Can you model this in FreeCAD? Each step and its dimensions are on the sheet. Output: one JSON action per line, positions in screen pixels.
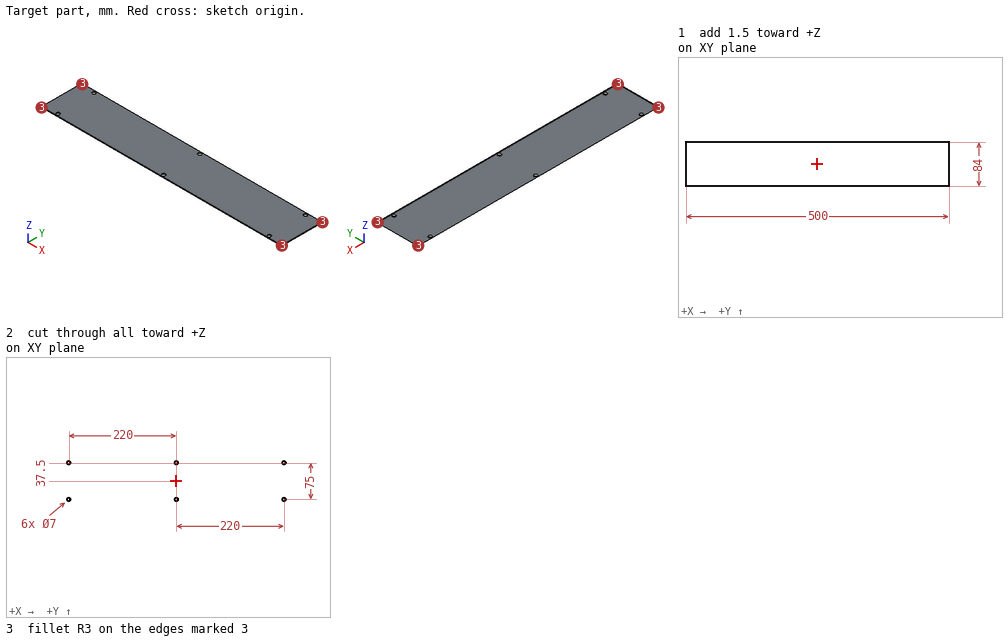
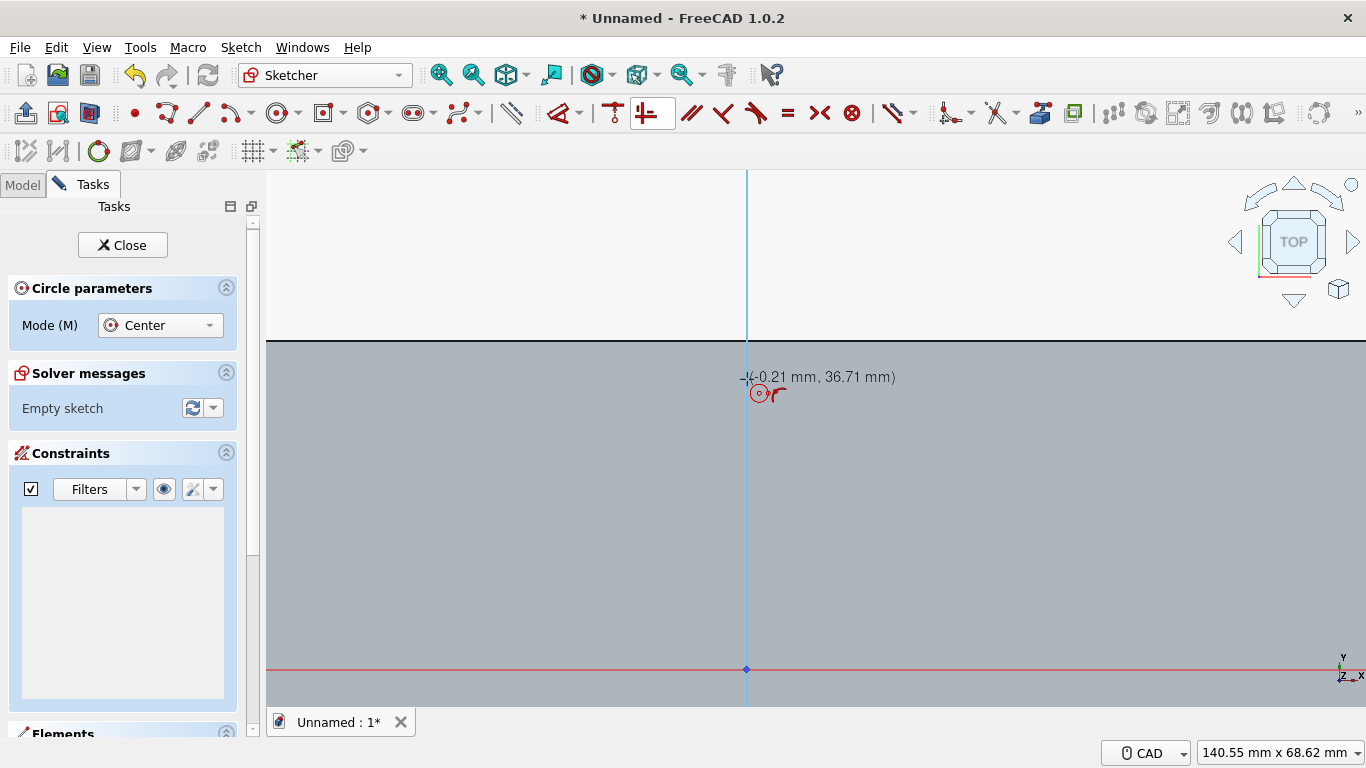
{"action": "scroll", "coordinate": [748, 380], "scroll_direction": "down", "scroll_amount": 8}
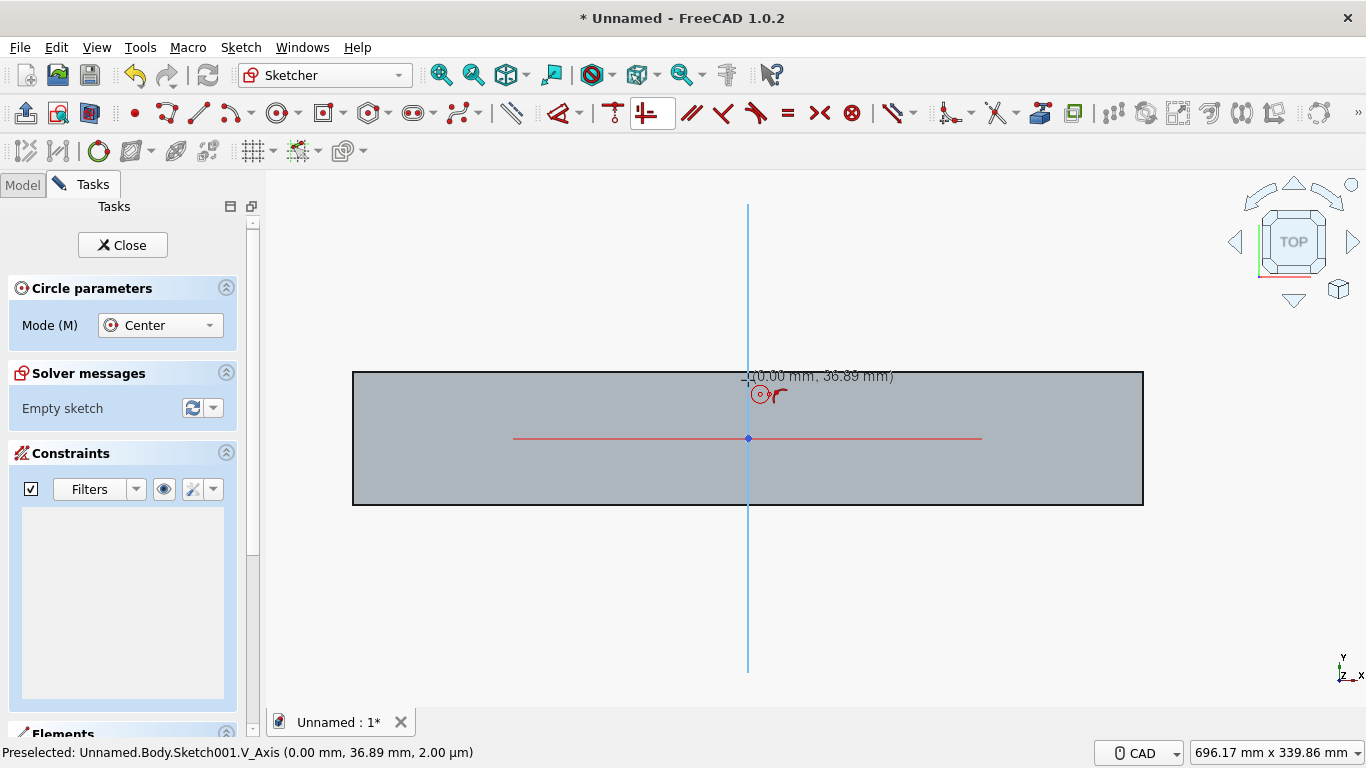
{"action": "left_click", "coordinate": [748, 380]}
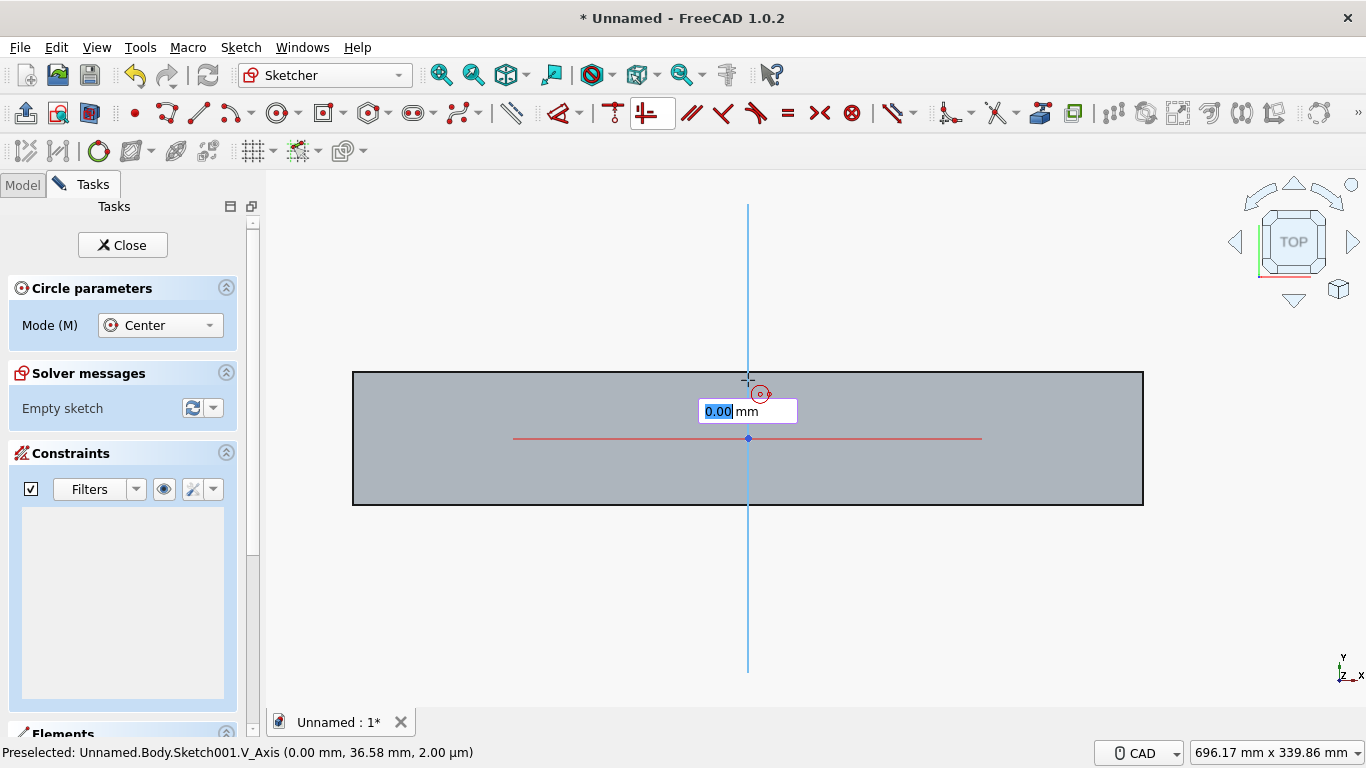
{"action": "scroll", "coordinate": [753, 378], "scroll_direction": "up", "scroll_amount": 6}
{"action": "mouse_move", "coordinate": [753, 376]}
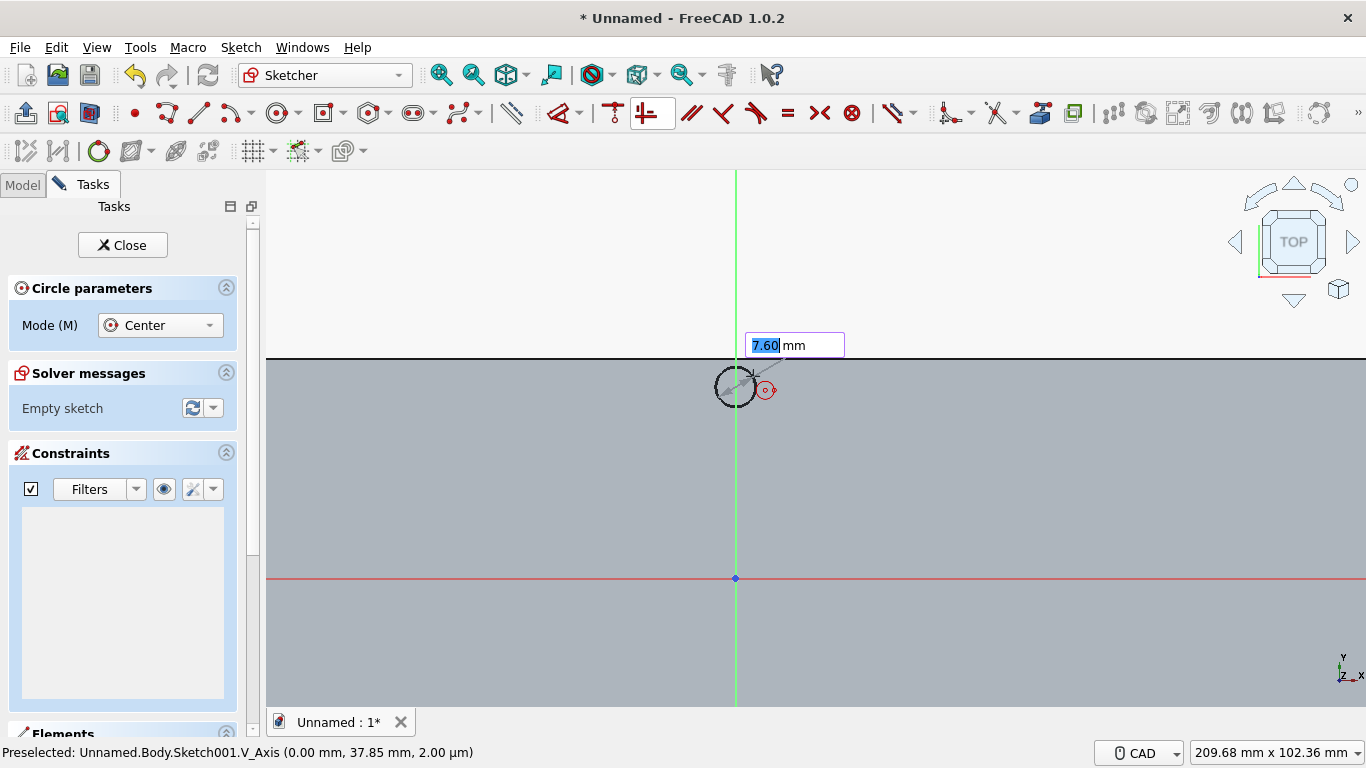
{"action": "type", "text": "7"}
{"action": "key", "text": "Return"}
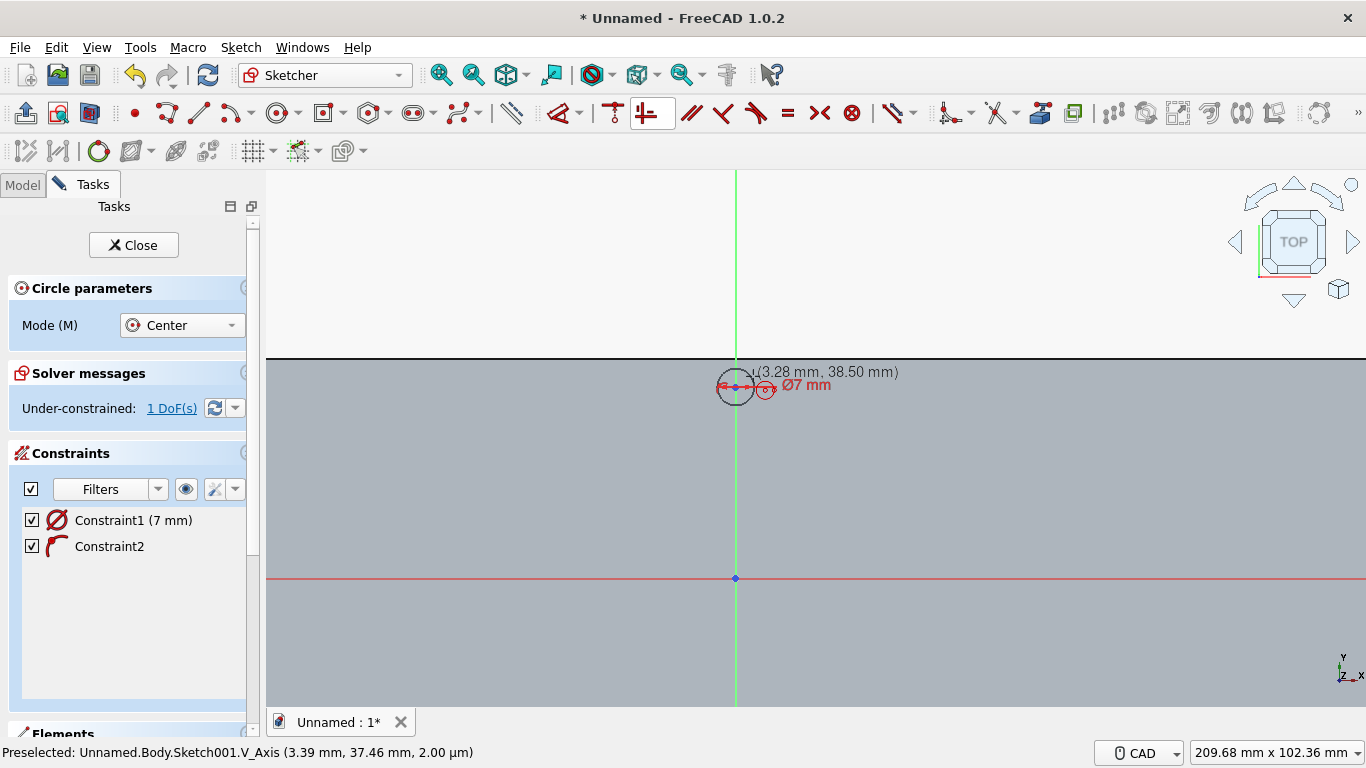
{"action": "scroll", "coordinate": [753, 378], "scroll_direction": "down", "scroll_amount": 6}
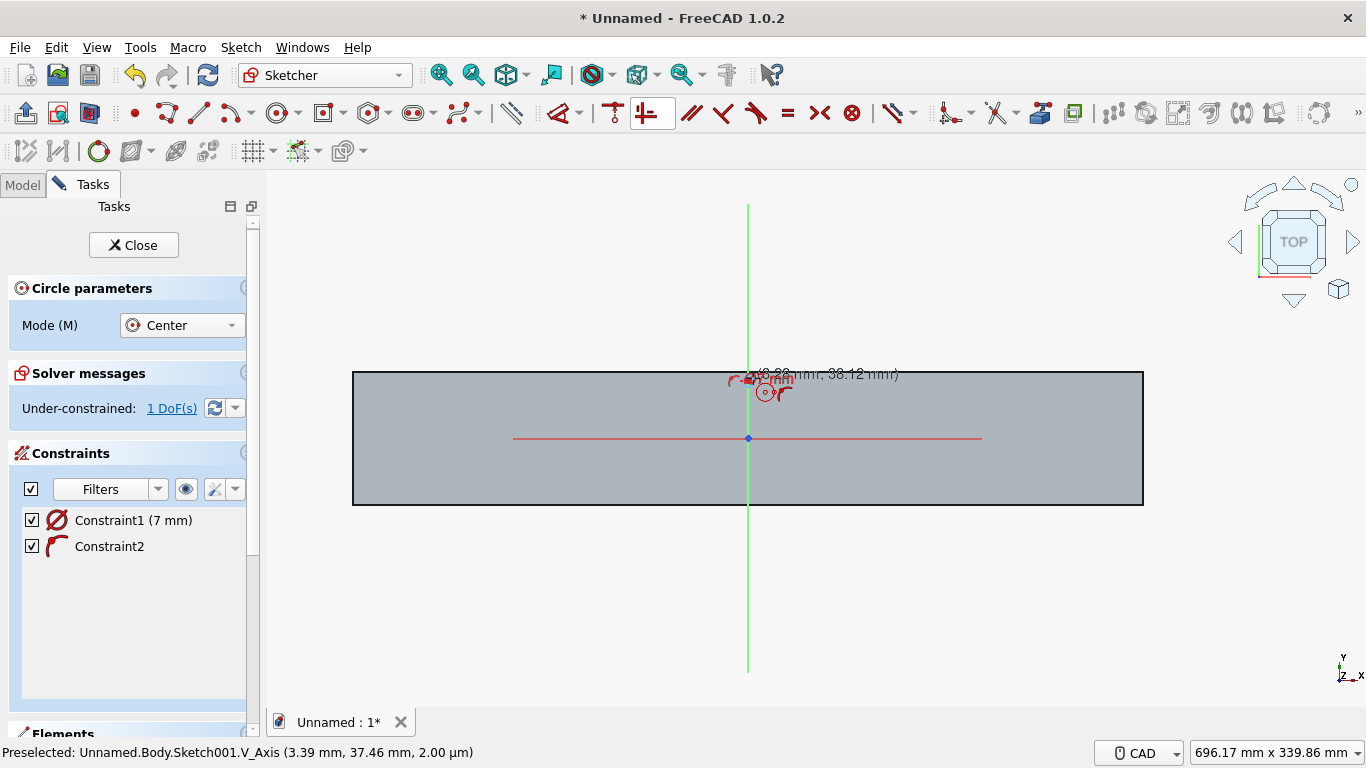
{"action": "scroll", "coordinate": [401, 380], "scroll_direction": "up", "scroll_amount": 8}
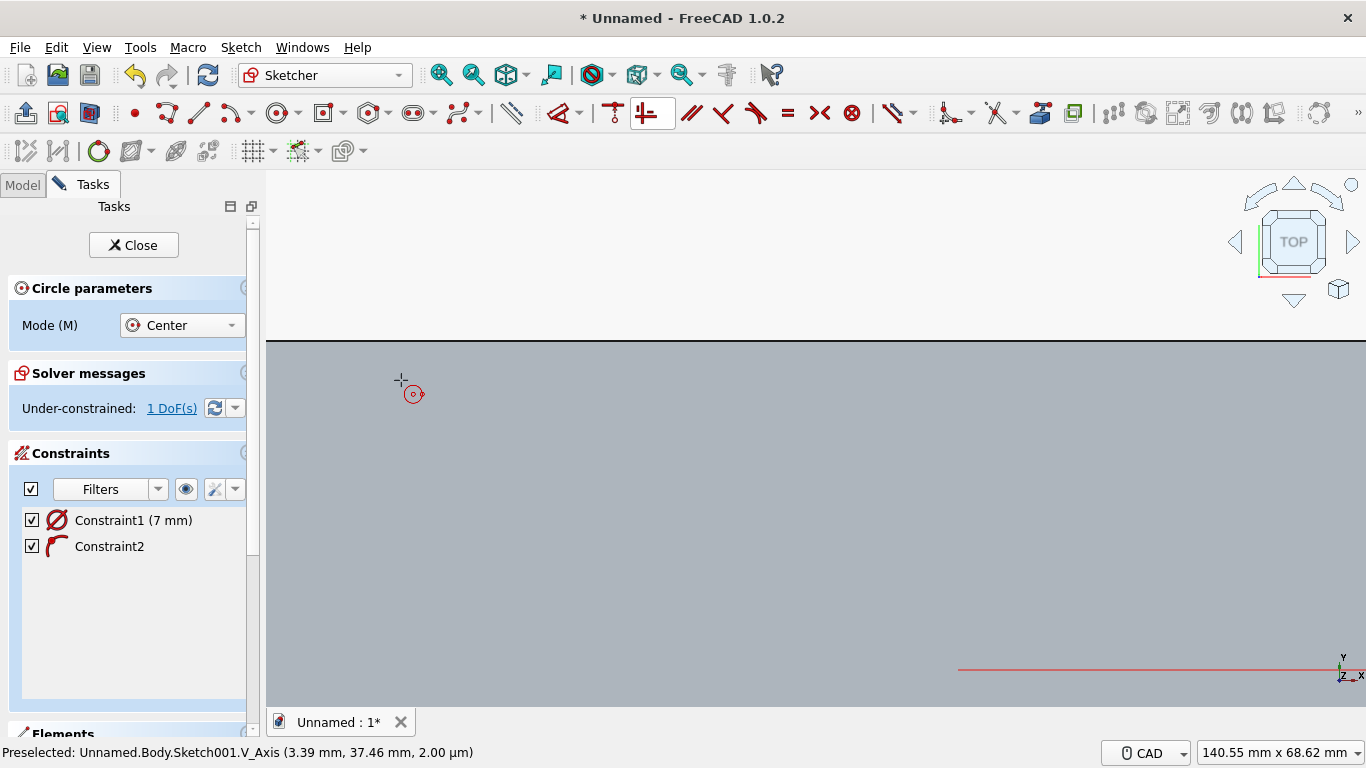
{"action": "scroll", "coordinate": [400, 380], "scroll_direction": "down", "scroll_amount": 8}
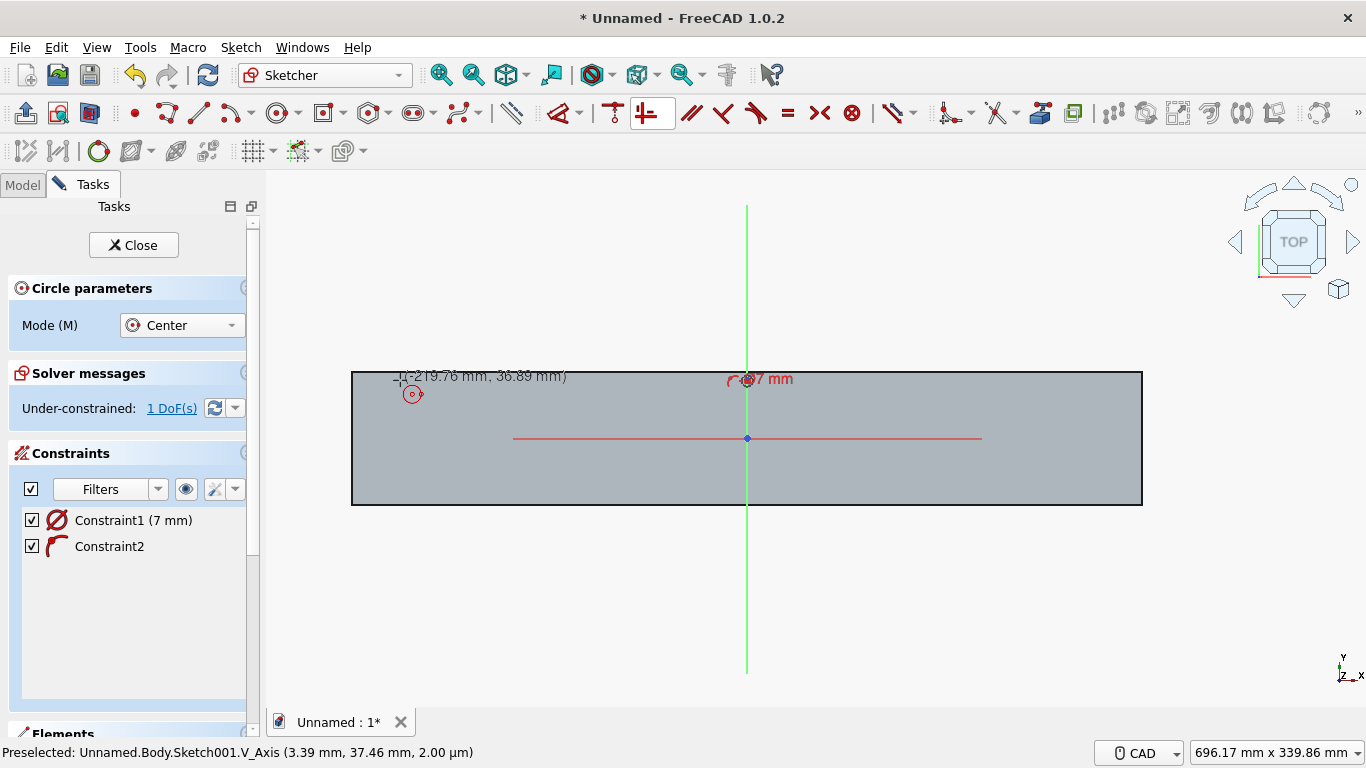
{"action": "left_click", "coordinate": [400, 380]}
{"action": "mouse_move", "coordinate": [404, 376]}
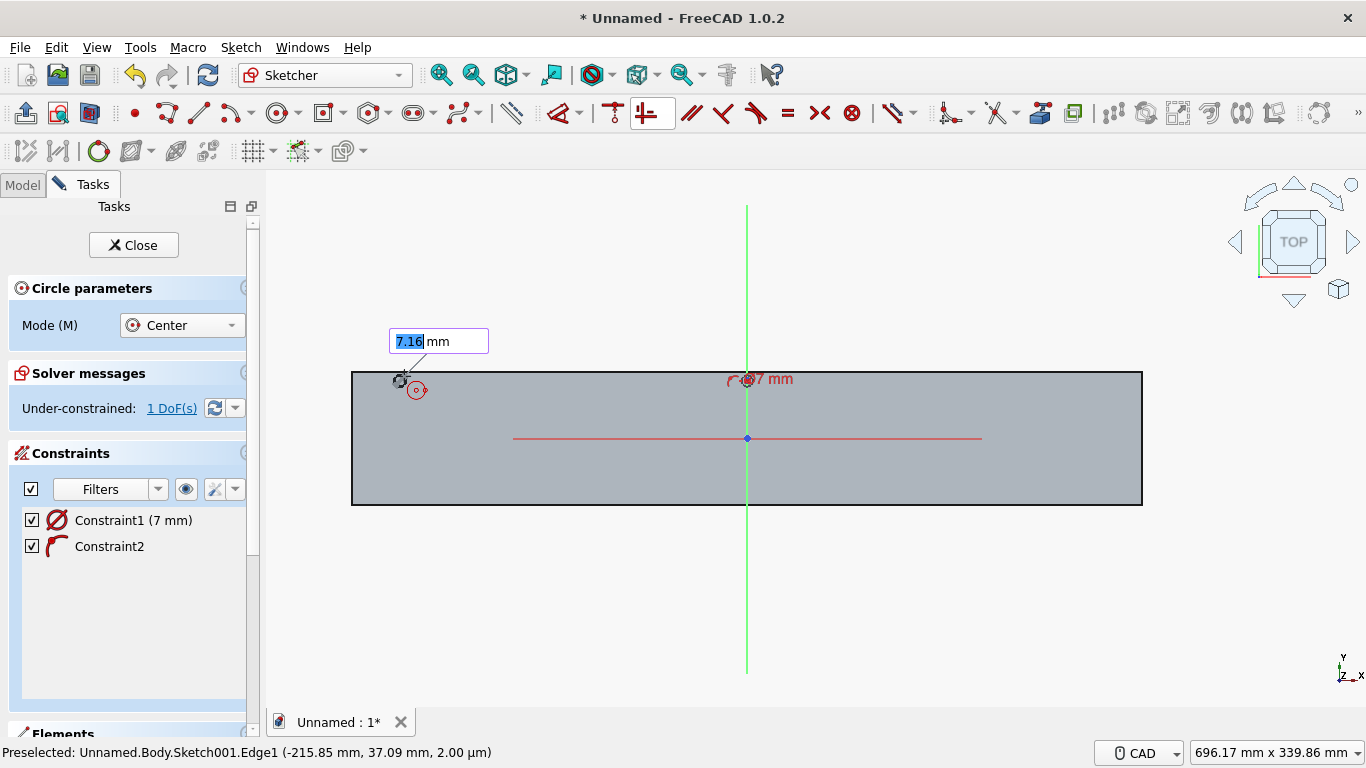
{"action": "type", "text": "7"}
{"action": "key", "text": "Return"}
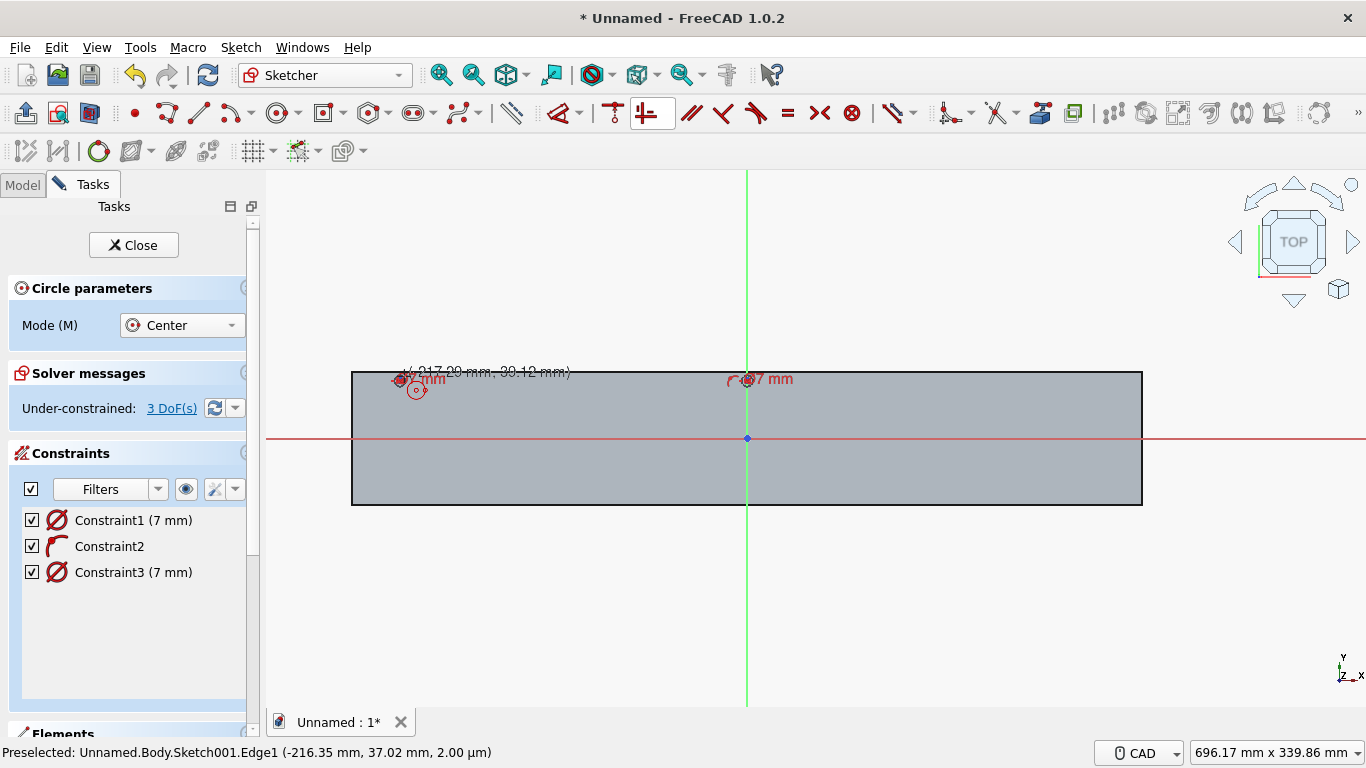
{"action": "scroll", "coordinate": [1095, 498], "scroll_direction": "up", "scroll_amount": 8}